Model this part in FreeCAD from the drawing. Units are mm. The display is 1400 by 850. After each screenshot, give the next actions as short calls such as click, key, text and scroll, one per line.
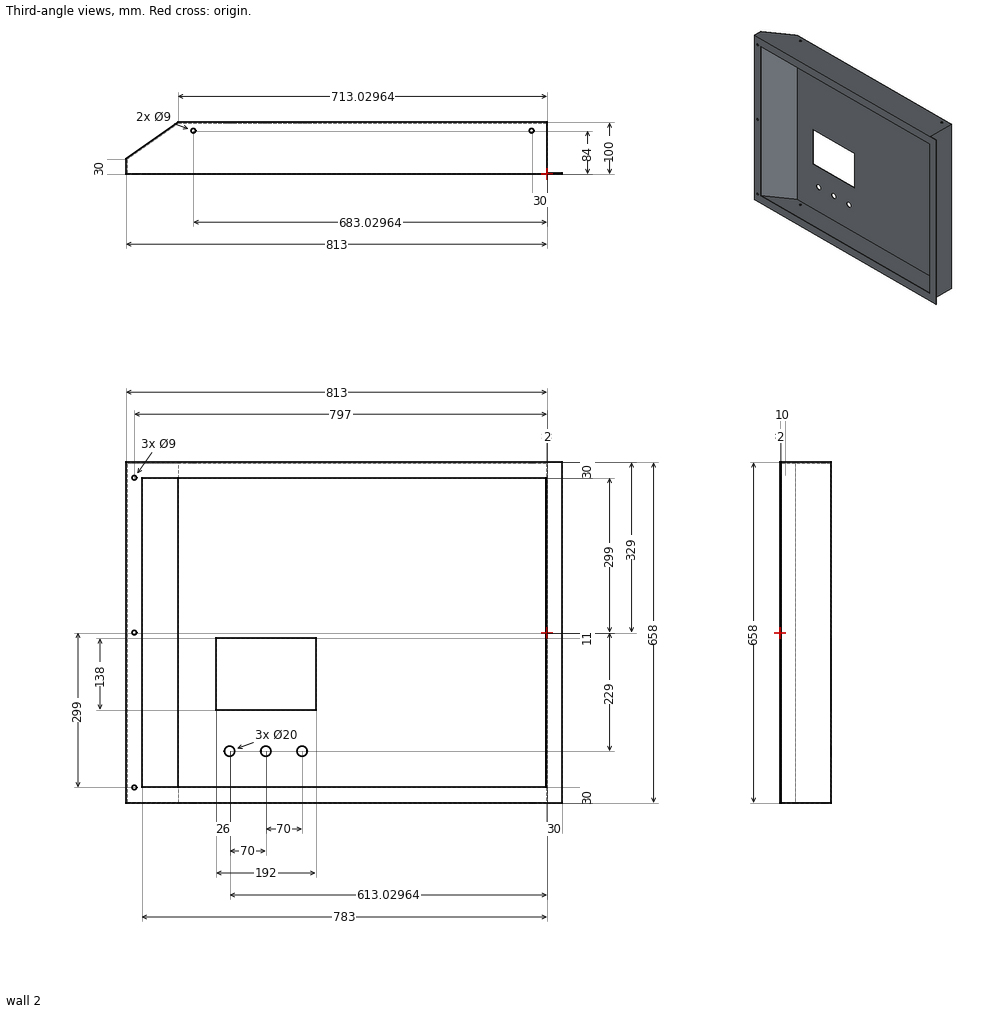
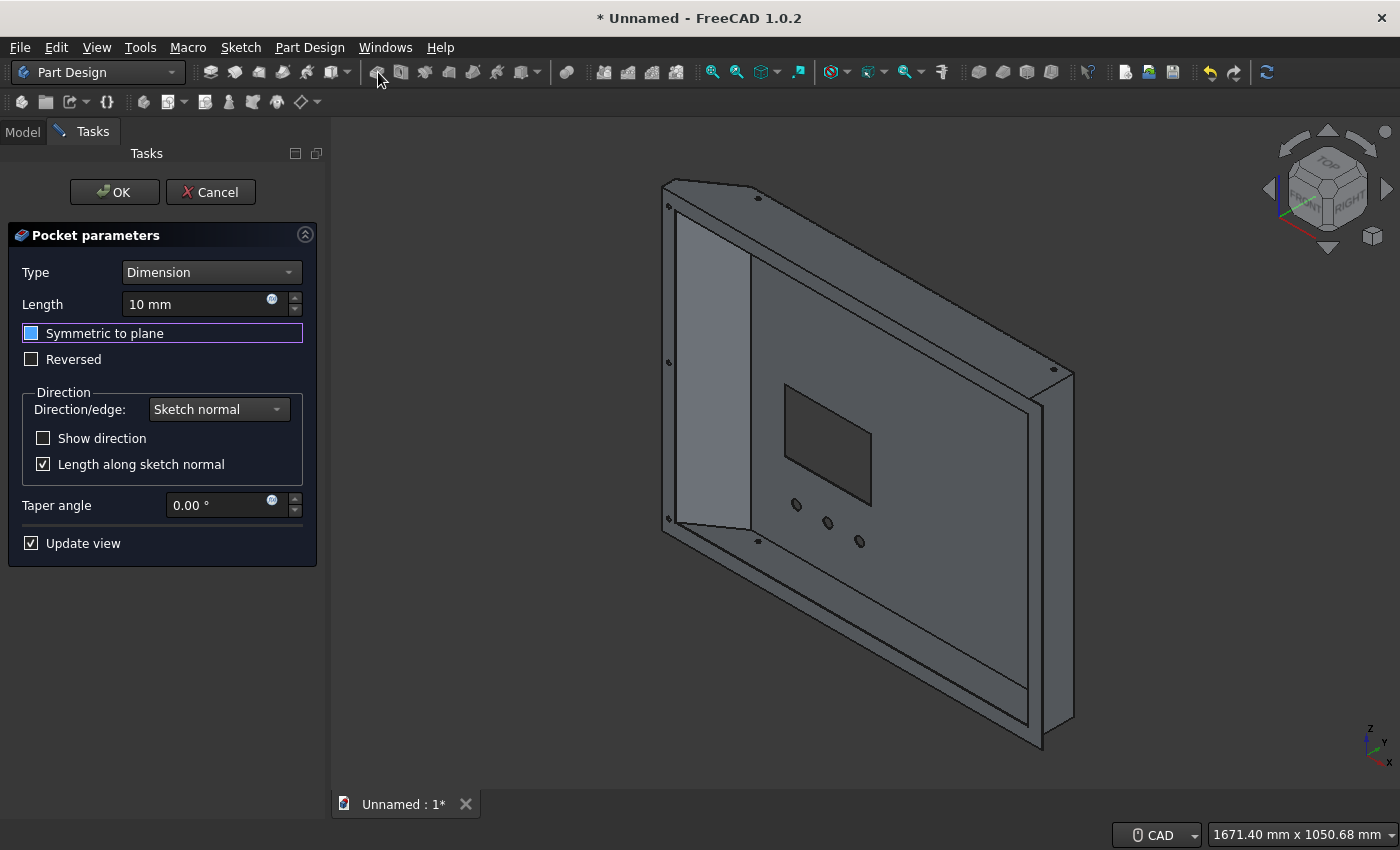
click(115, 192)